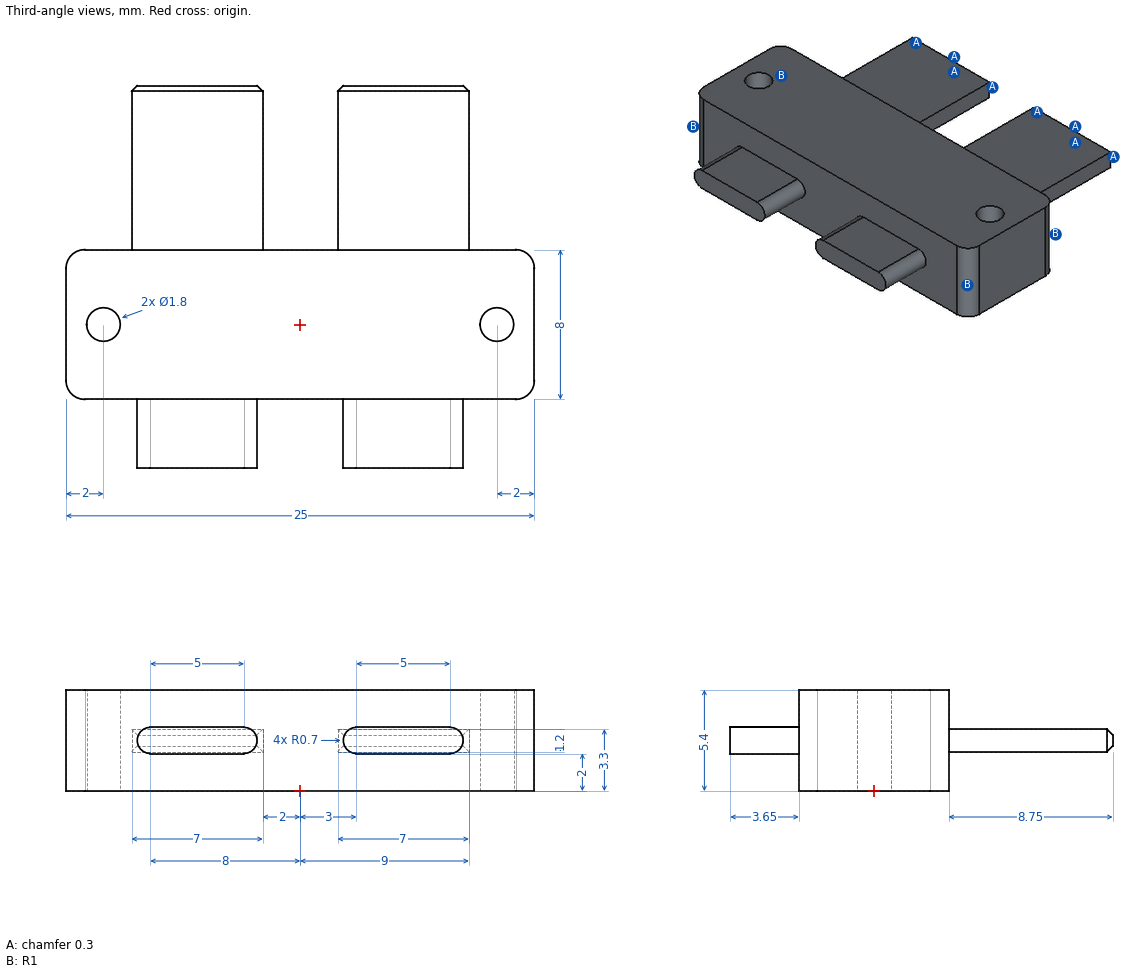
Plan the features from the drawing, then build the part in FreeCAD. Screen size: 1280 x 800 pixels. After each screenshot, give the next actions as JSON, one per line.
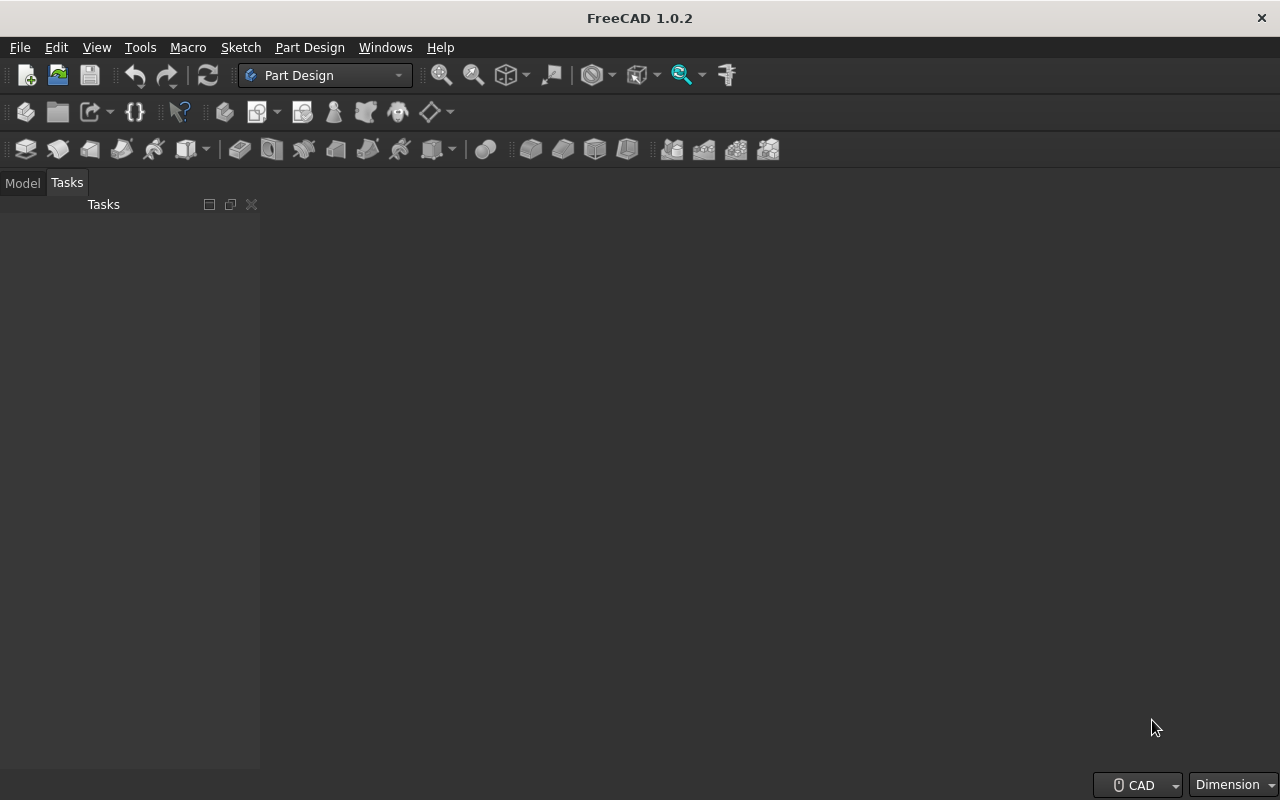
{"action": "left_click", "coordinate": [26, 76]}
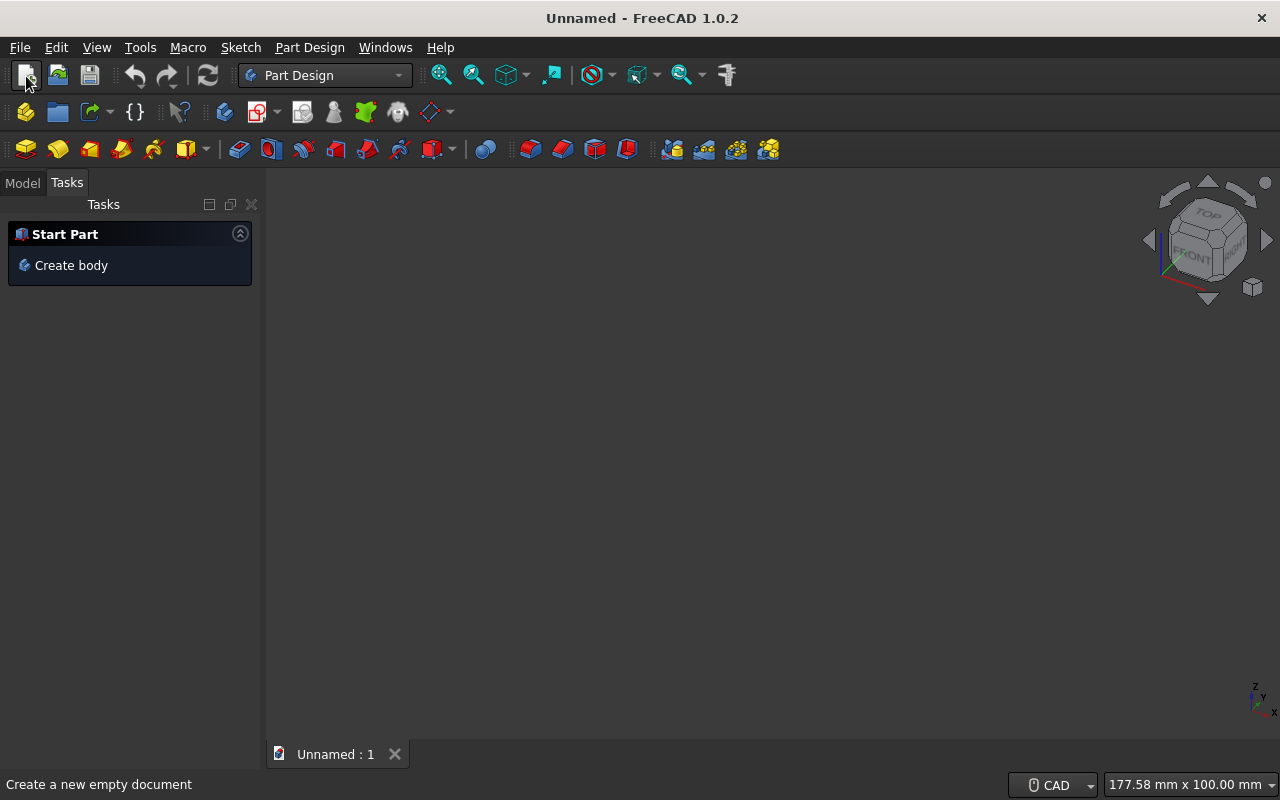
{"action": "left_click", "coordinate": [258, 112]}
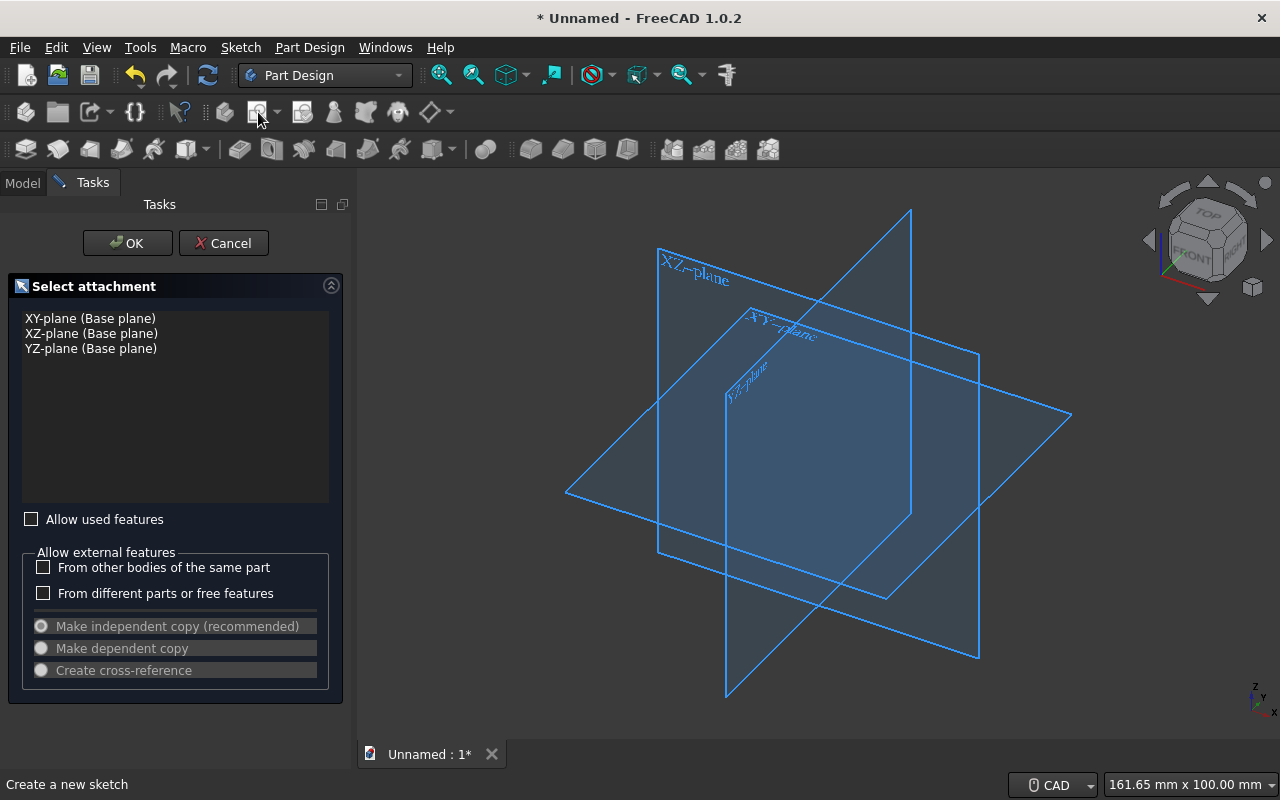
{"action": "left_click", "coordinate": [82, 318]}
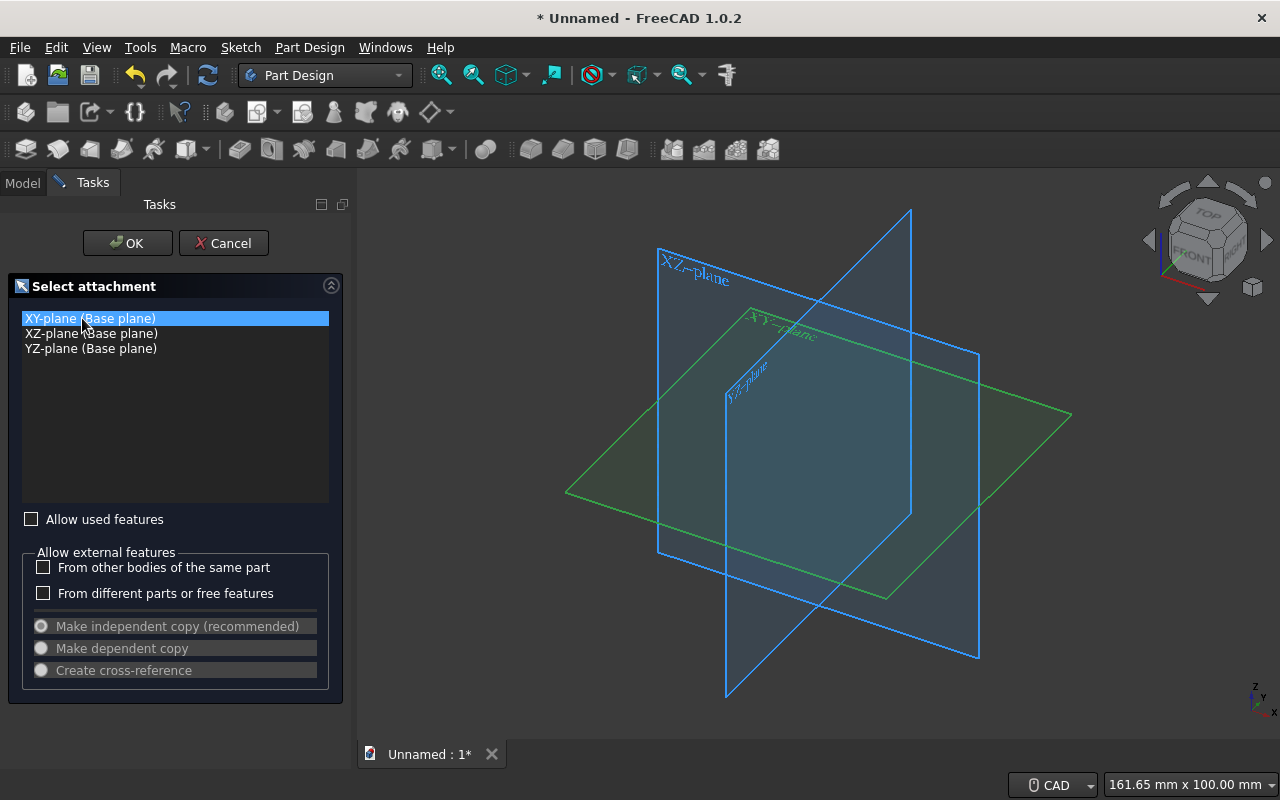
{"action": "left_click", "coordinate": [128, 243]}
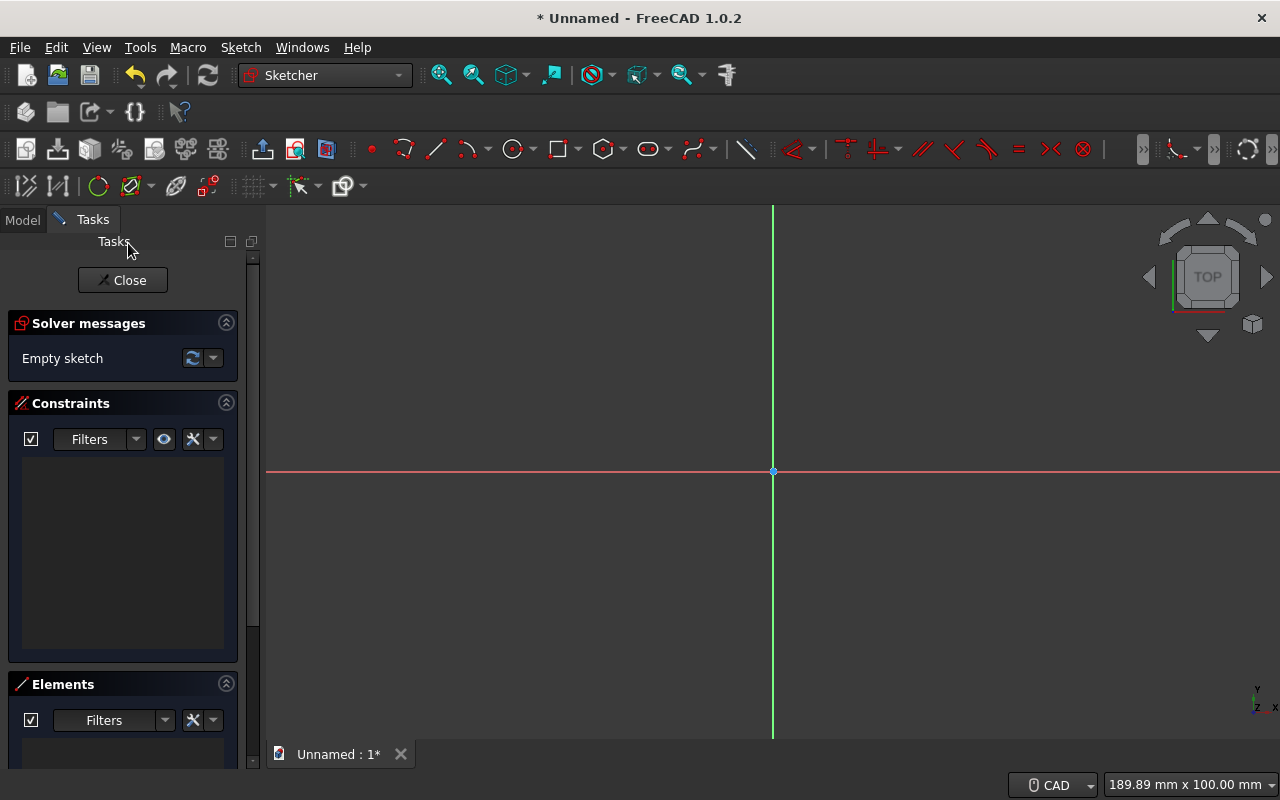
{"action": "scroll", "coordinate": [795, 472], "scroll_direction": "up", "scroll_amount": 7}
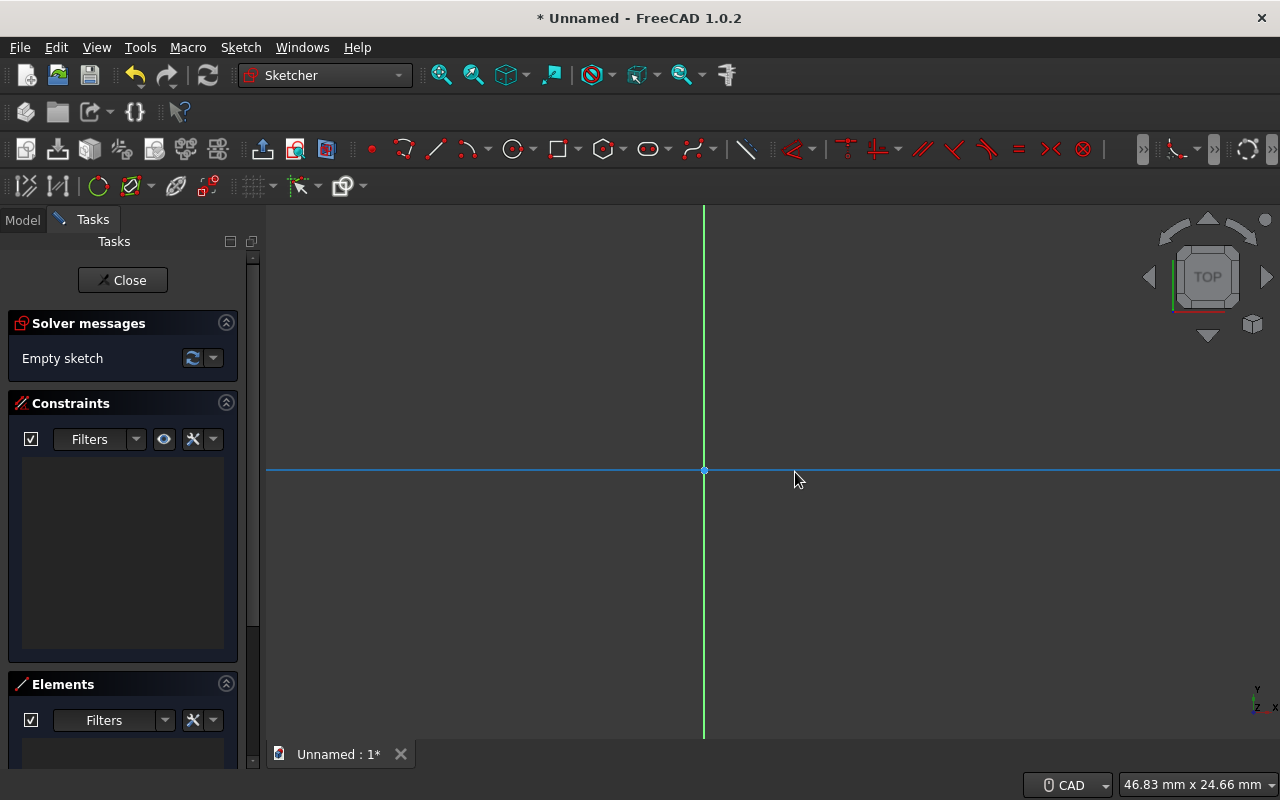
{"action": "left_click", "coordinate": [580, 150]}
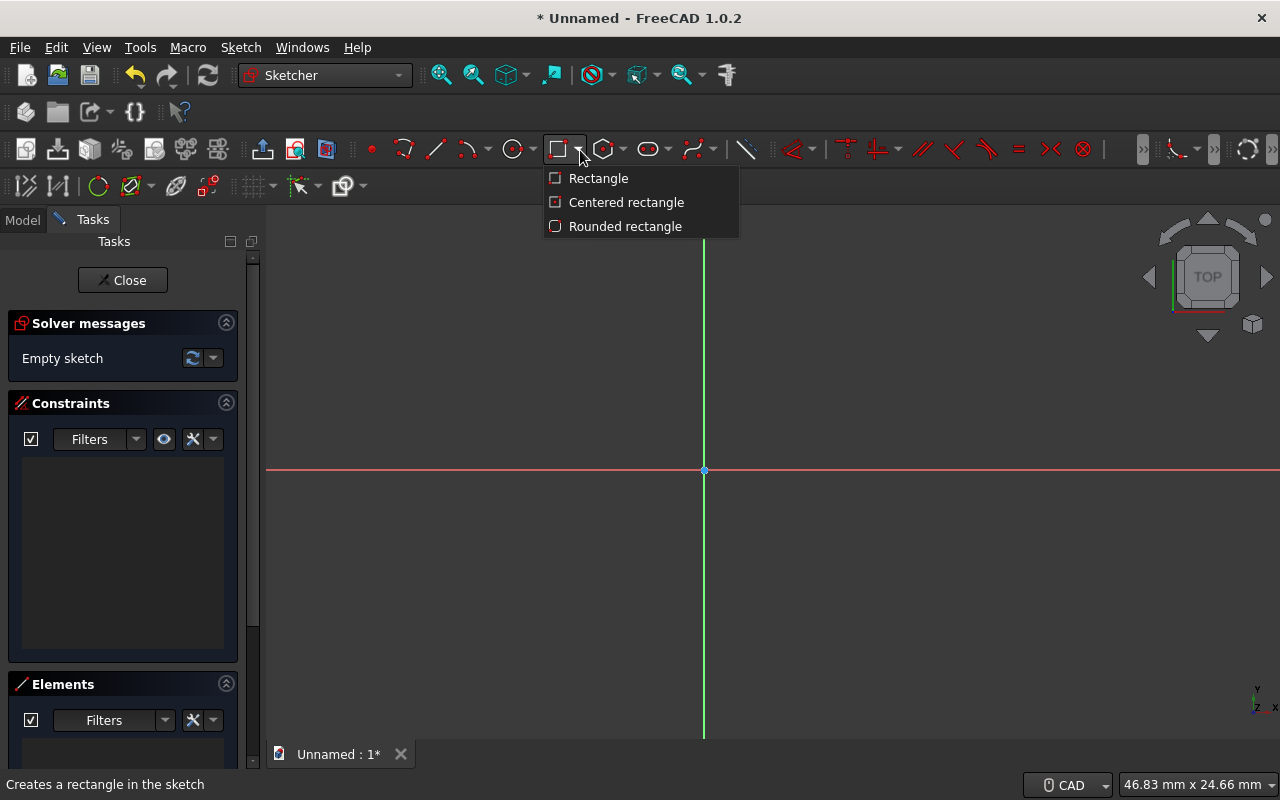
{"action": "left_click", "coordinate": [642, 202]}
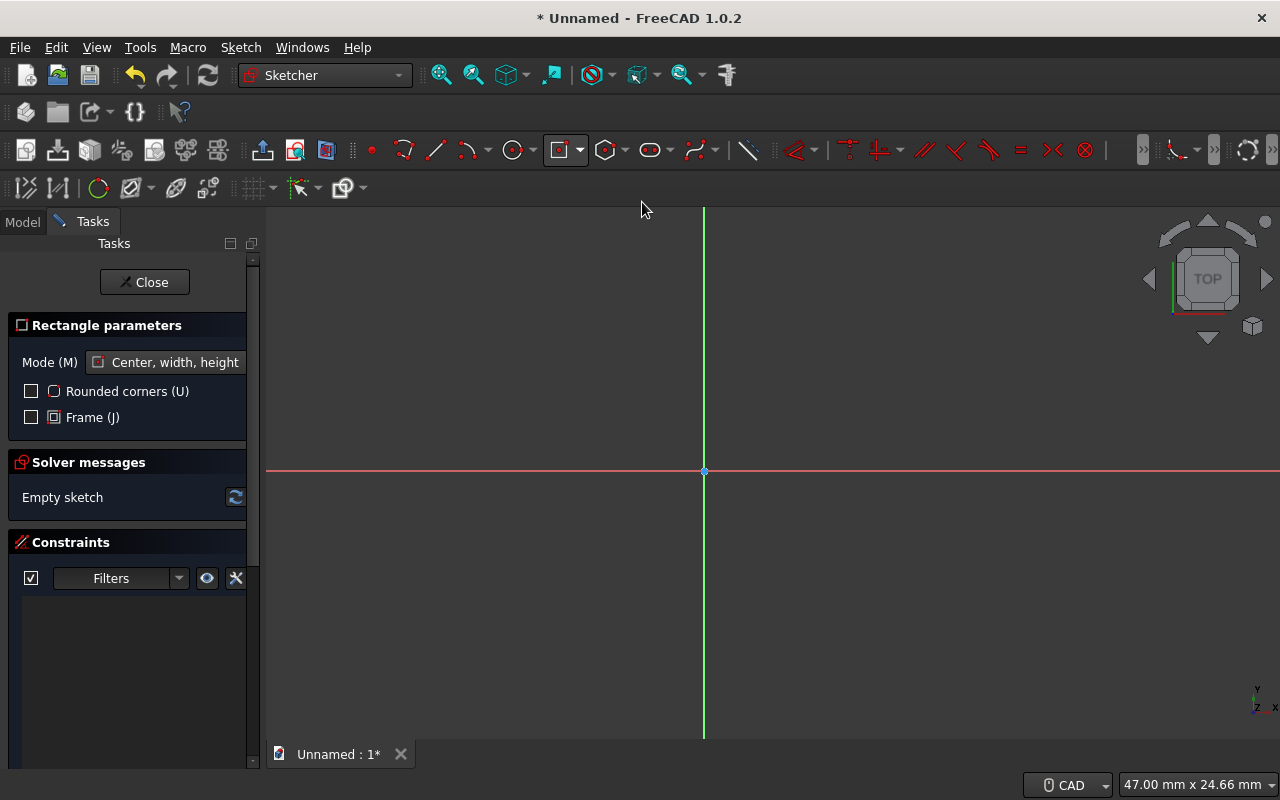
{"action": "left_click", "coordinate": [704, 471]}
{"action": "mouse_move", "coordinate": [974, 385]}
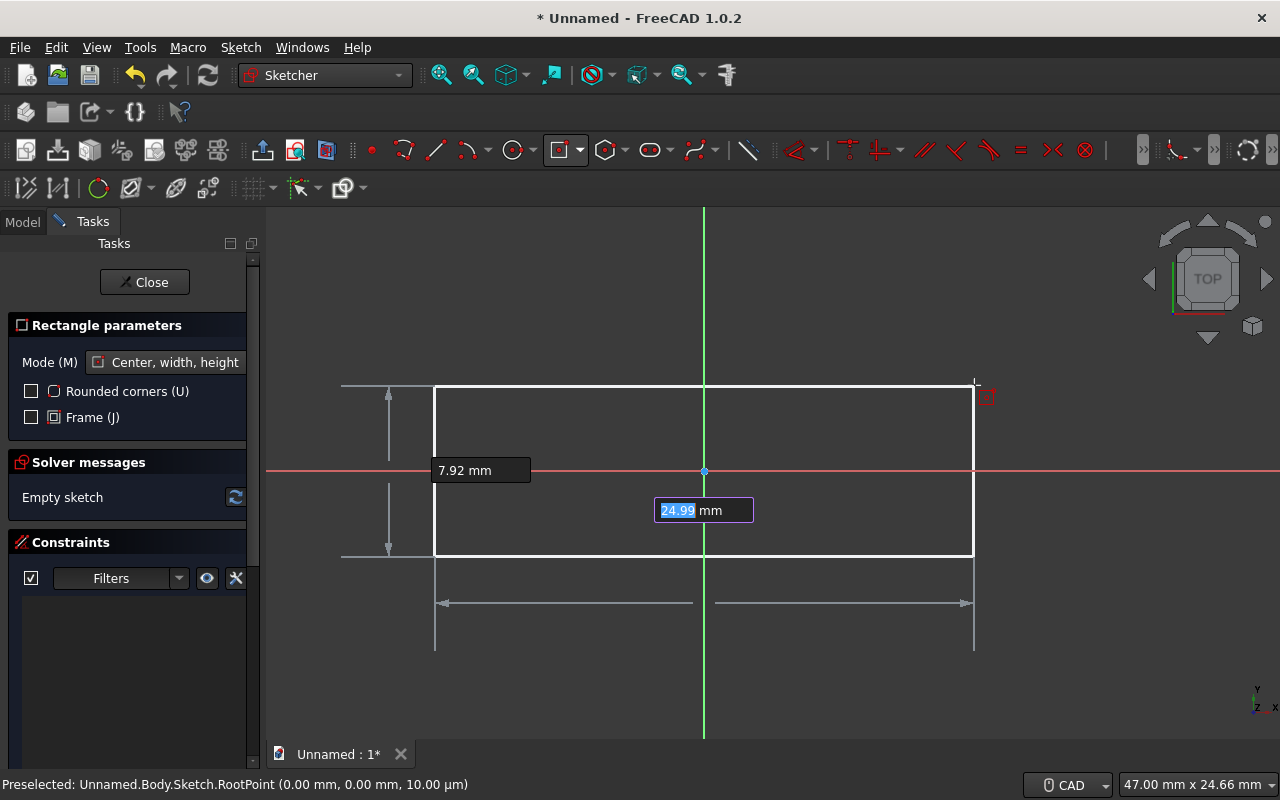
{"action": "type", "text": "25"}
{"action": "key", "text": "Tab"}
{"action": "type", "text": "8"}
{"action": "key", "text": "Return"}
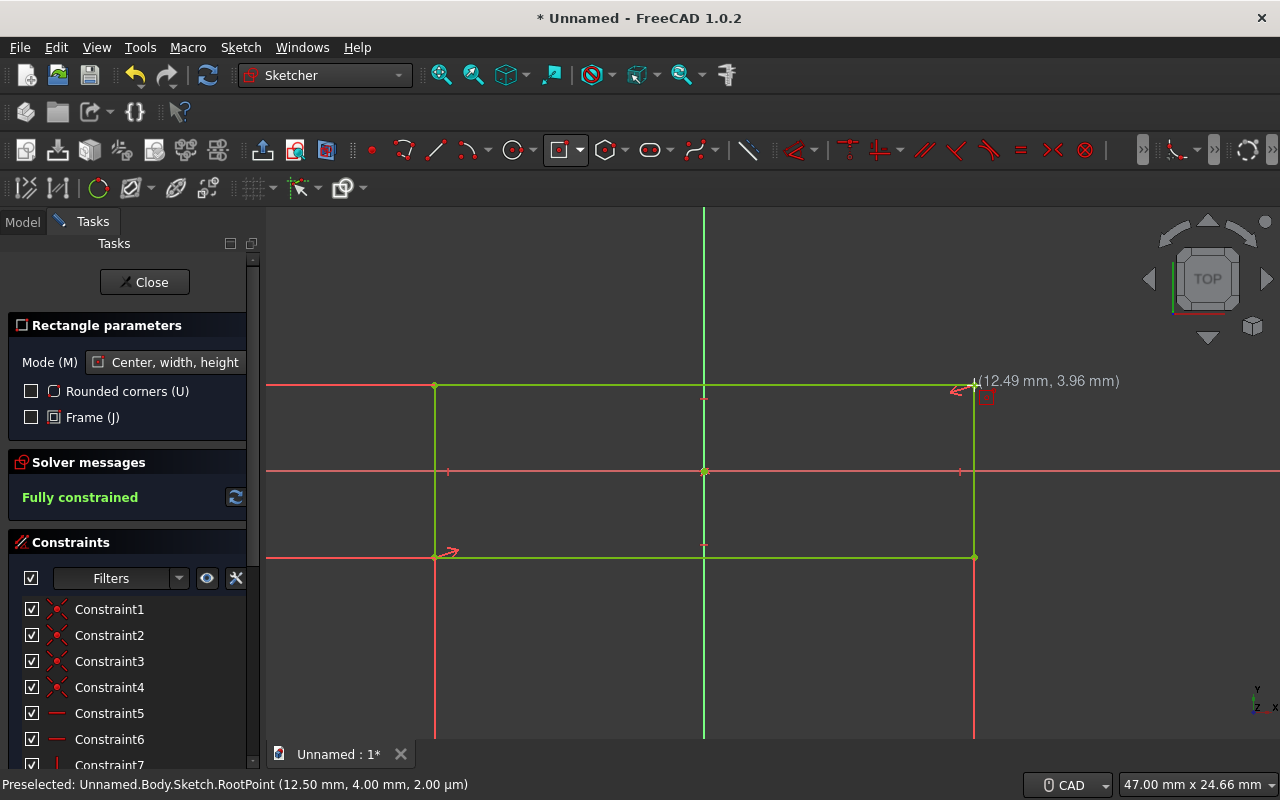
{"action": "left_click", "coordinate": [514, 150]}